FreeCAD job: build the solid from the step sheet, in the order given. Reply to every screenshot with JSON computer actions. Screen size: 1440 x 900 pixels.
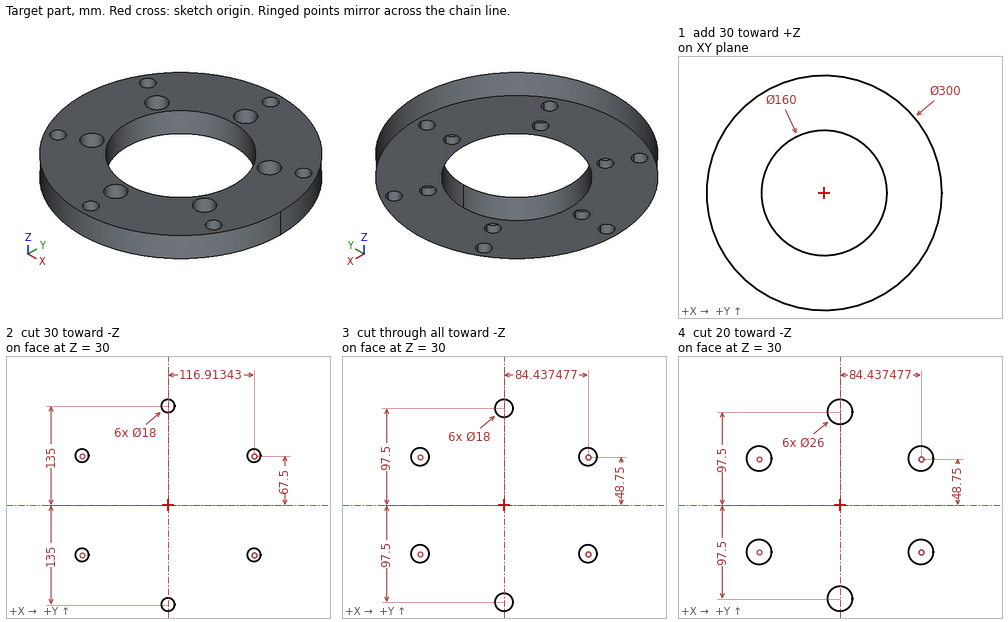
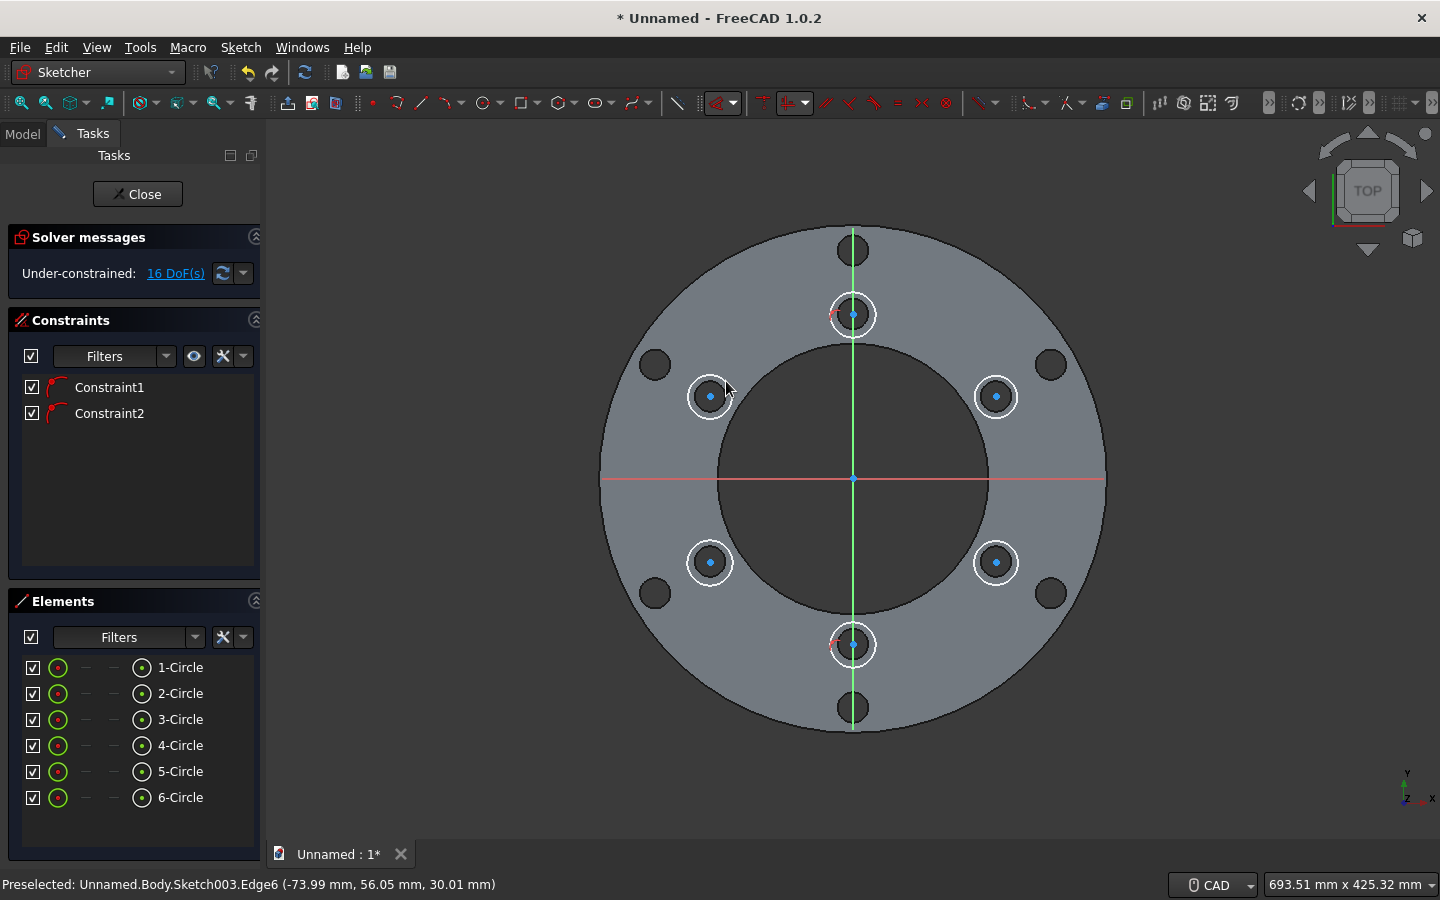
{"action": "left_click", "coordinate": [869, 299]}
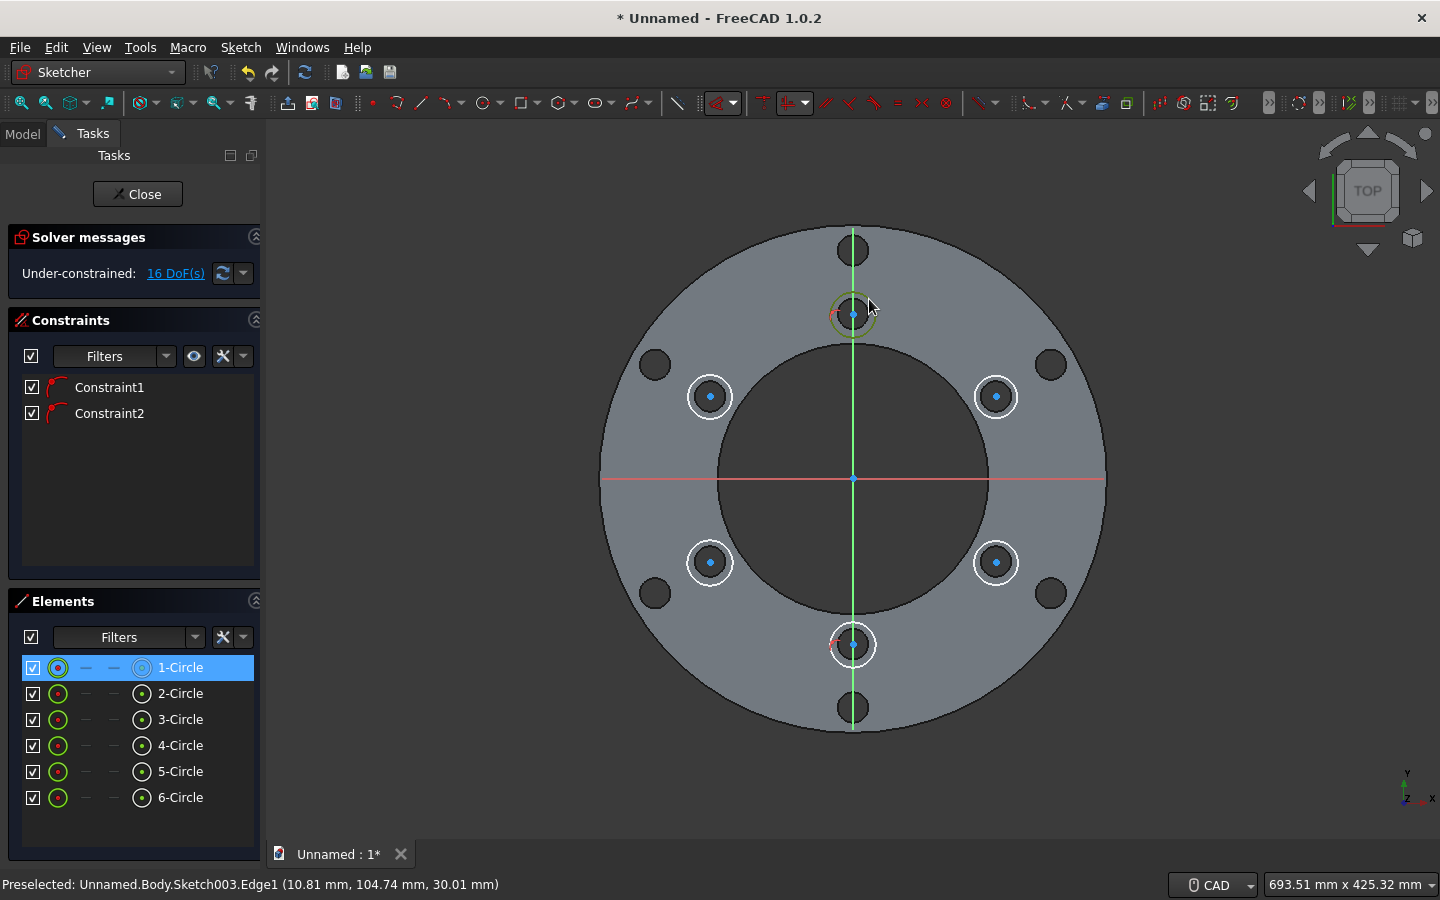
{"action": "left_click", "coordinate": [1011, 382]}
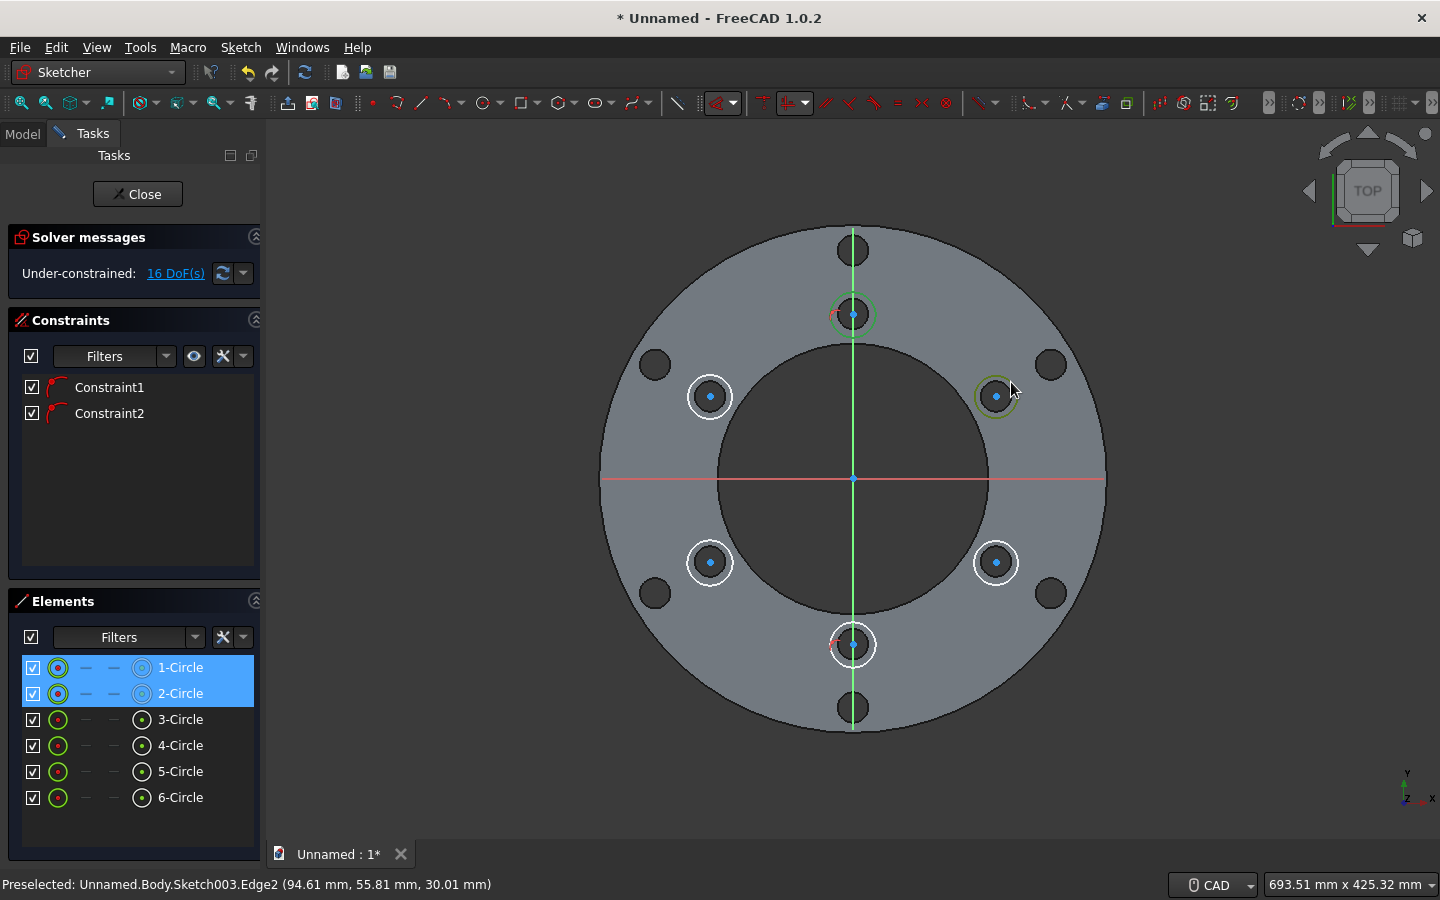
{"action": "left_click", "coordinate": [1011, 547]}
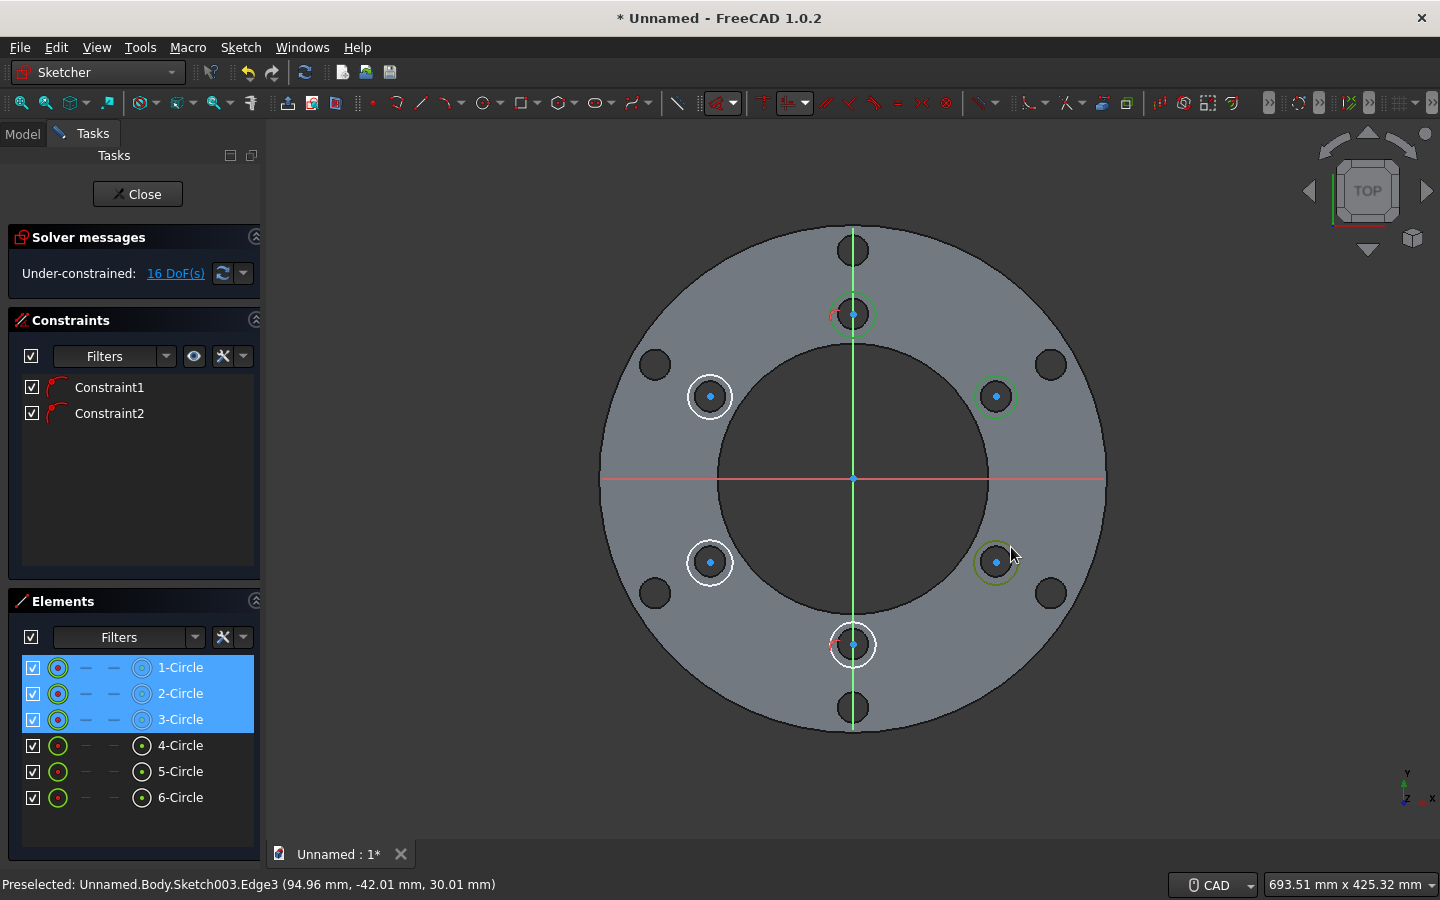
{"action": "left_click", "coordinate": [869, 629]}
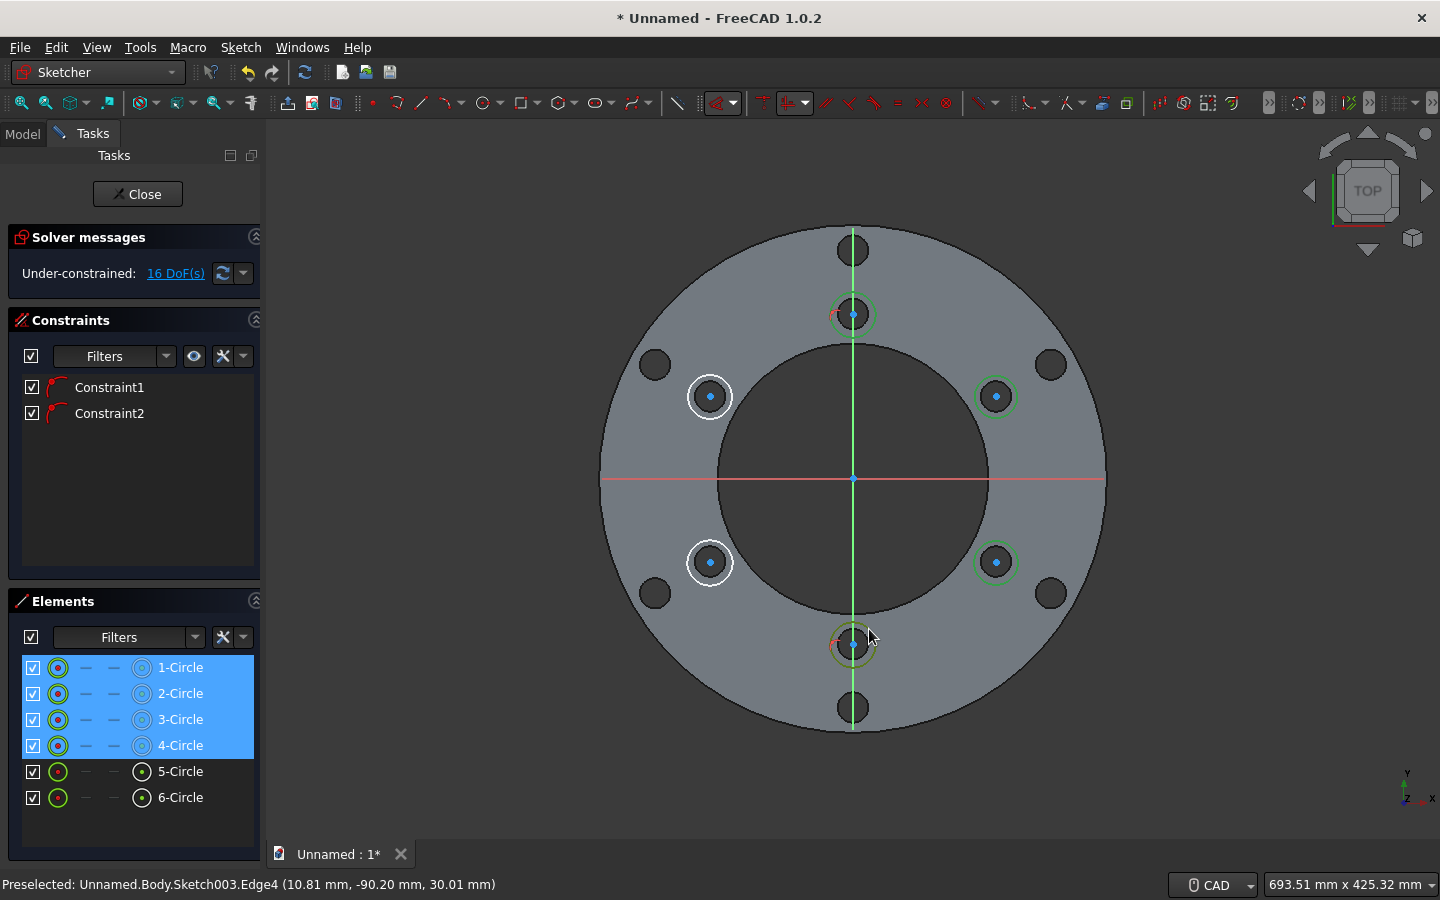
{"action": "left_click", "coordinate": [726, 547]}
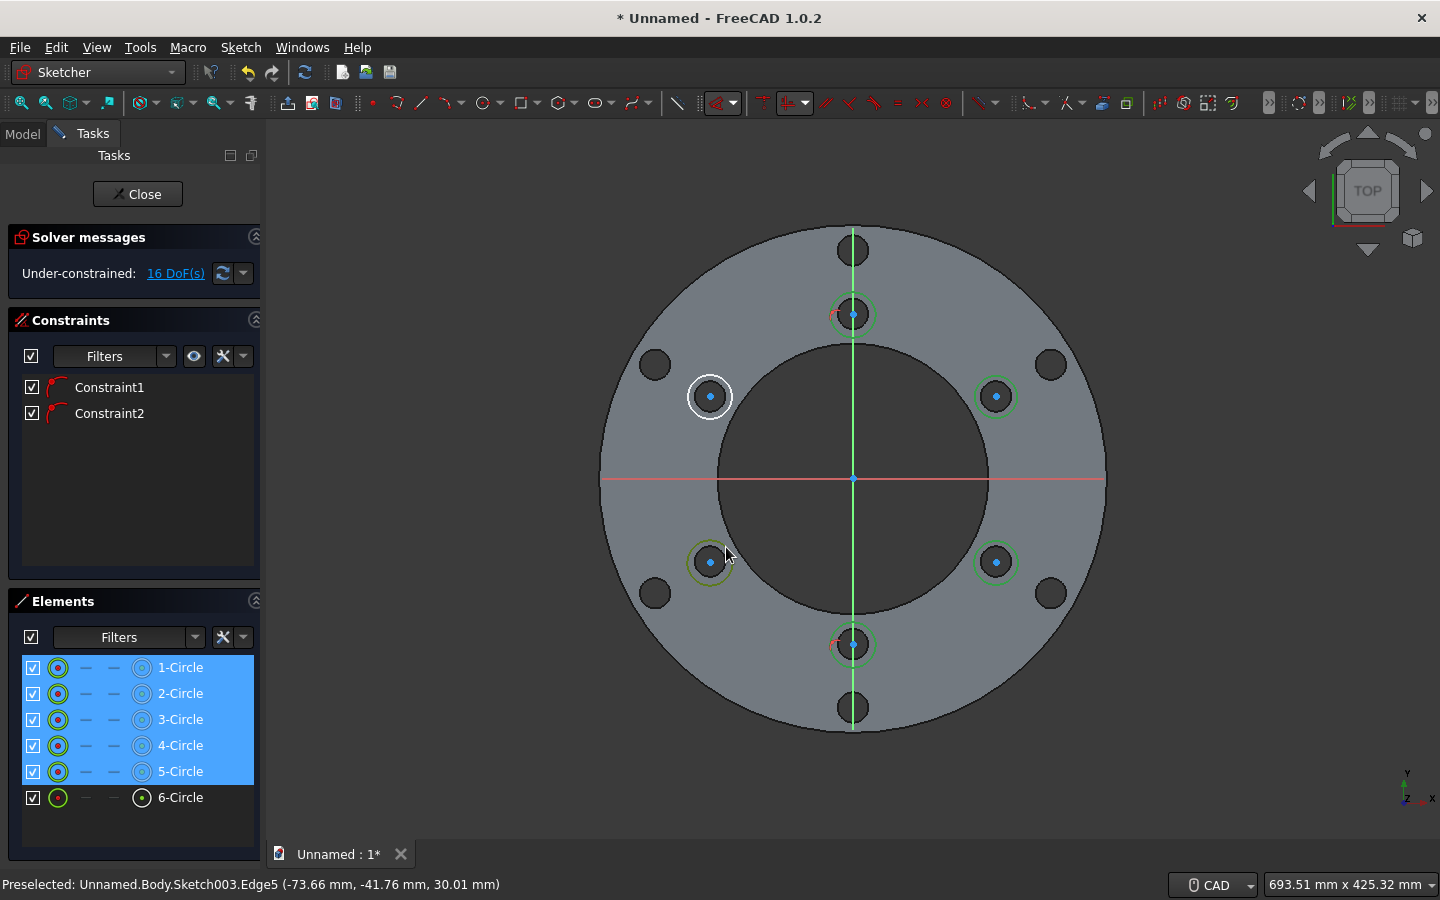
{"action": "left_click", "coordinate": [725, 381]}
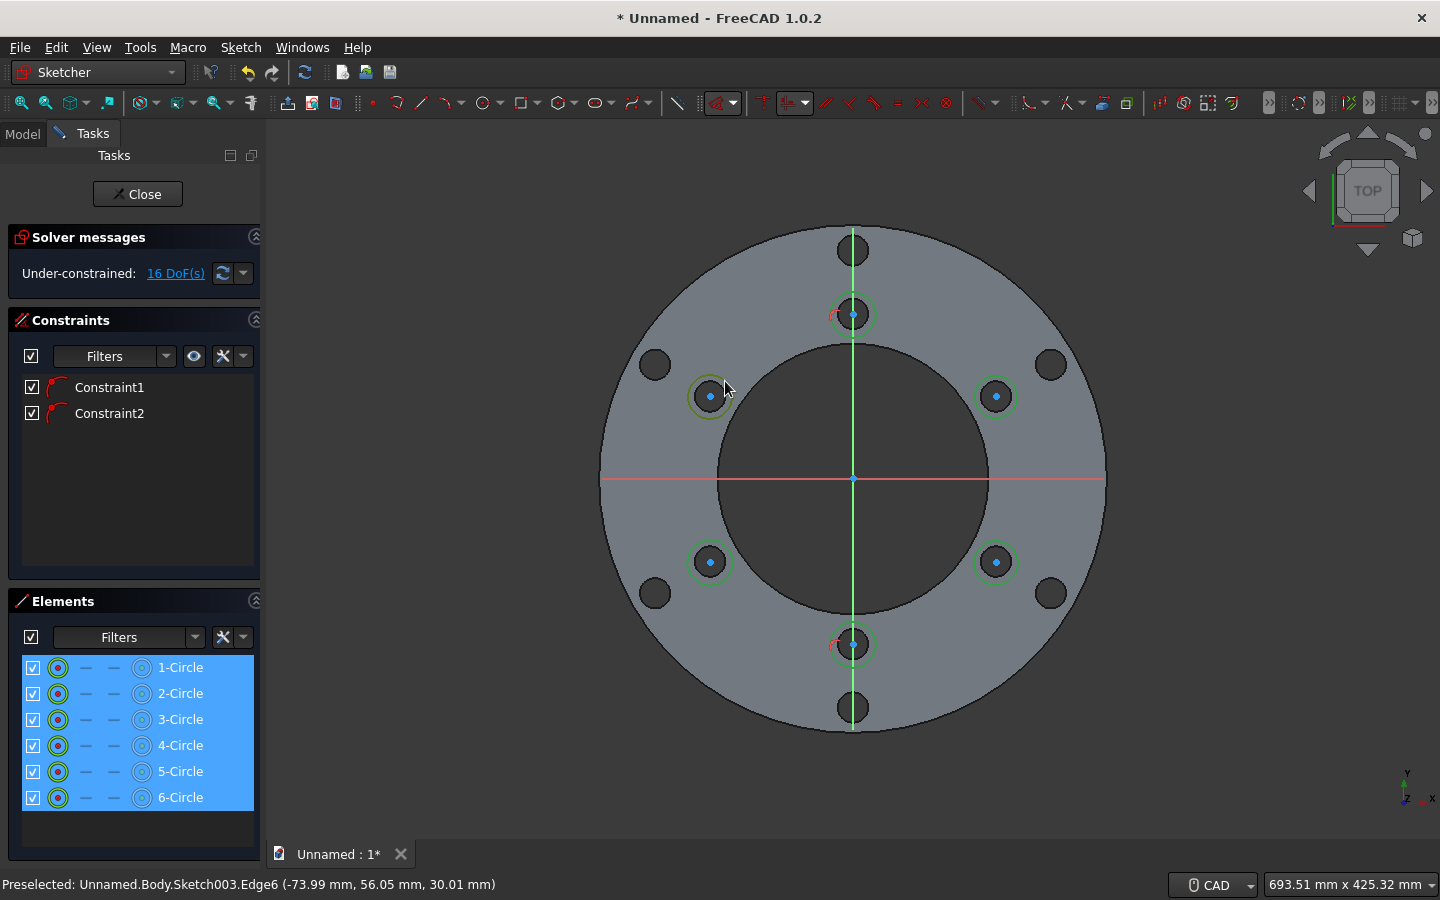
{"action": "key", "text": "e"}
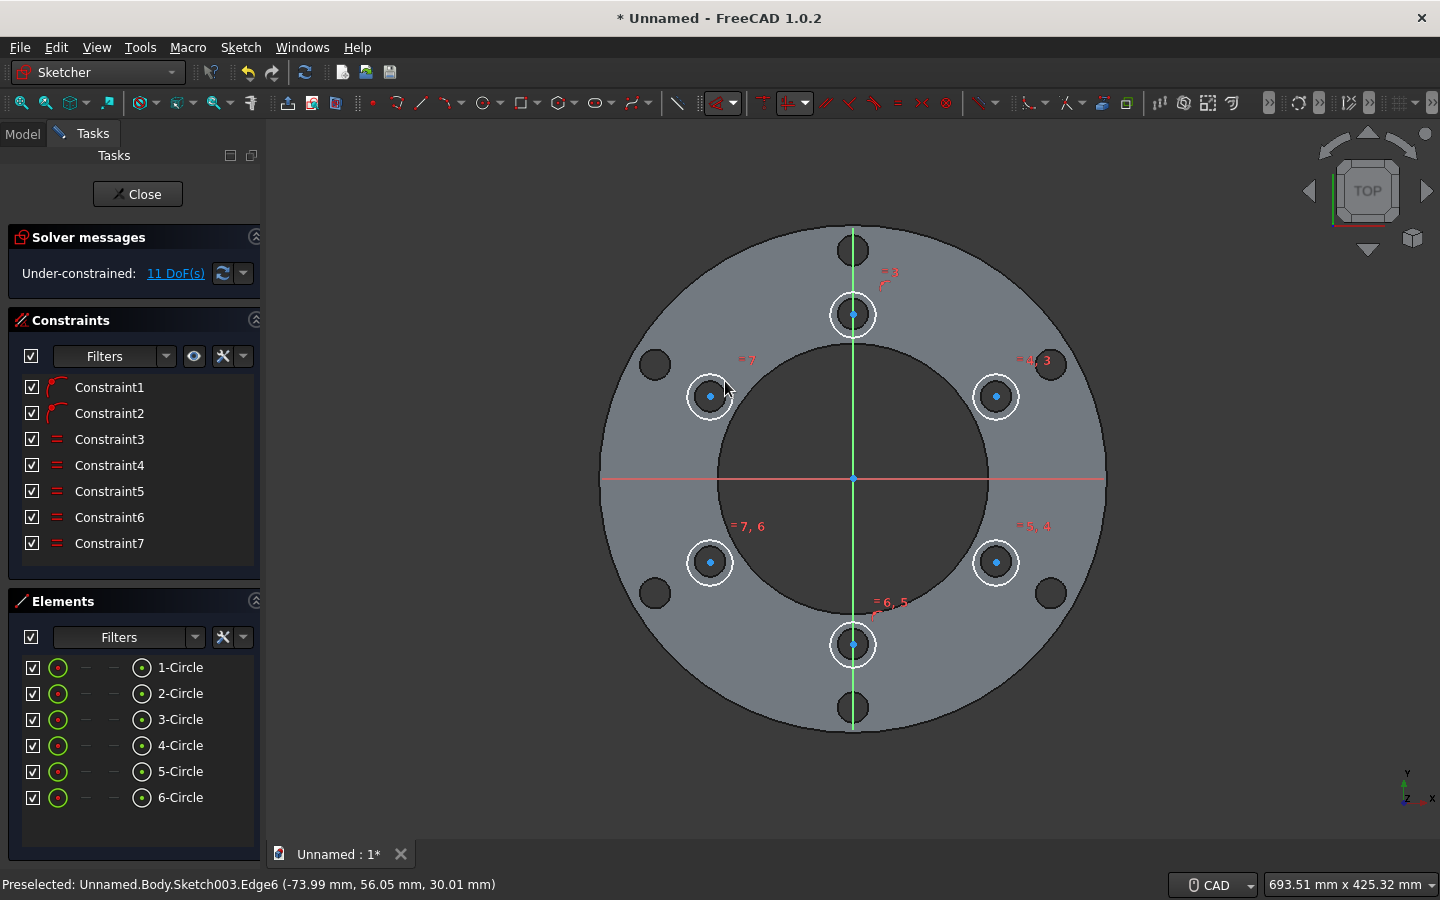
{"action": "left_click", "coordinate": [996, 397]}